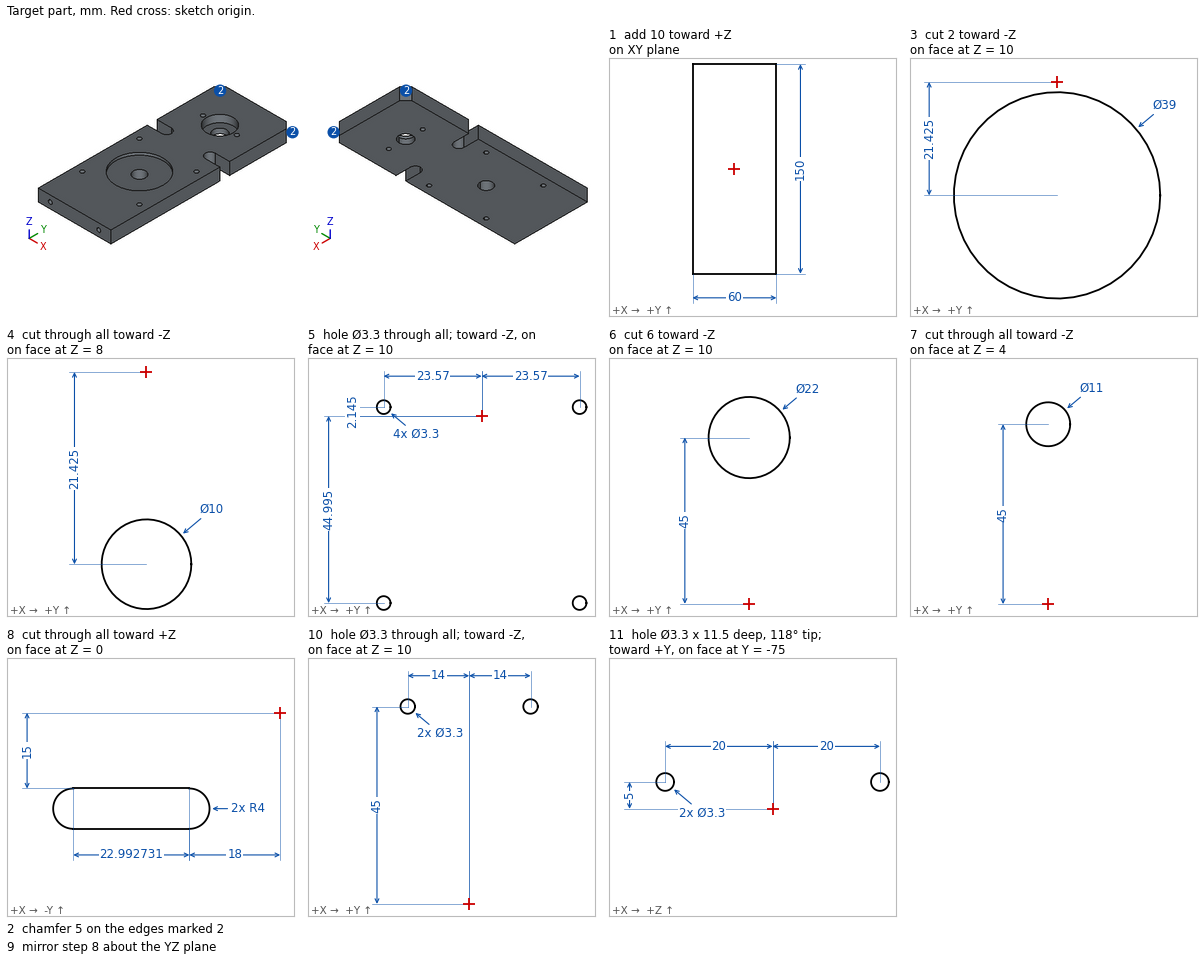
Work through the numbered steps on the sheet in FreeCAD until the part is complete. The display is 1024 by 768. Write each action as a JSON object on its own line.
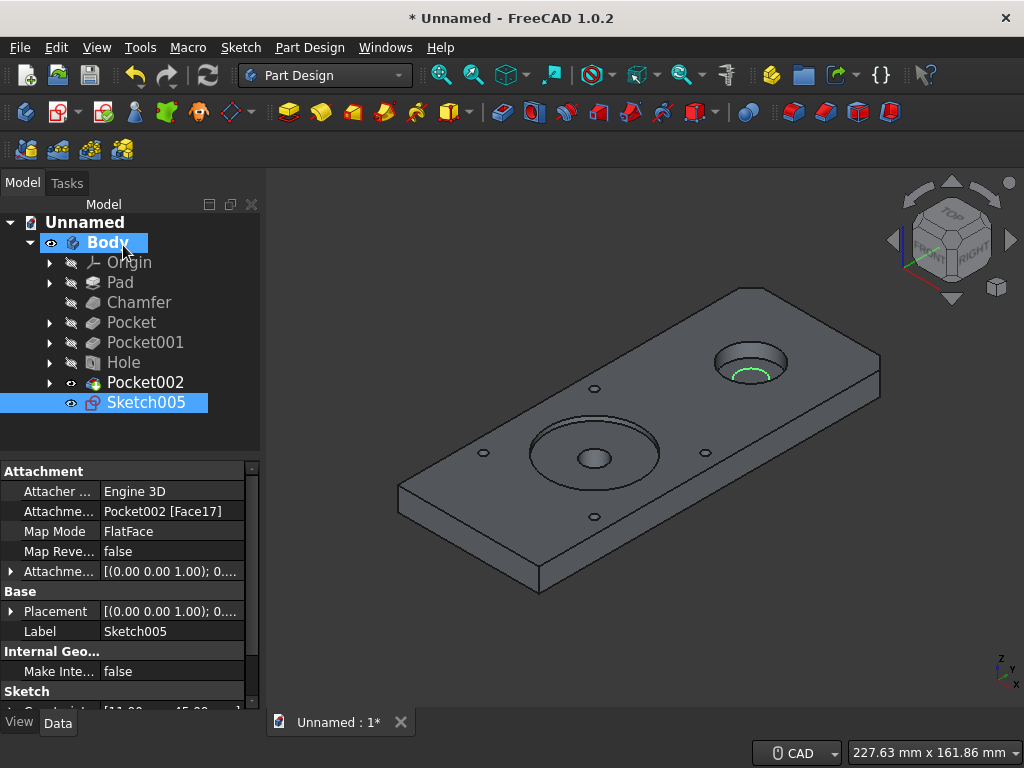
{"action": "left_click", "coordinate": [504, 112]}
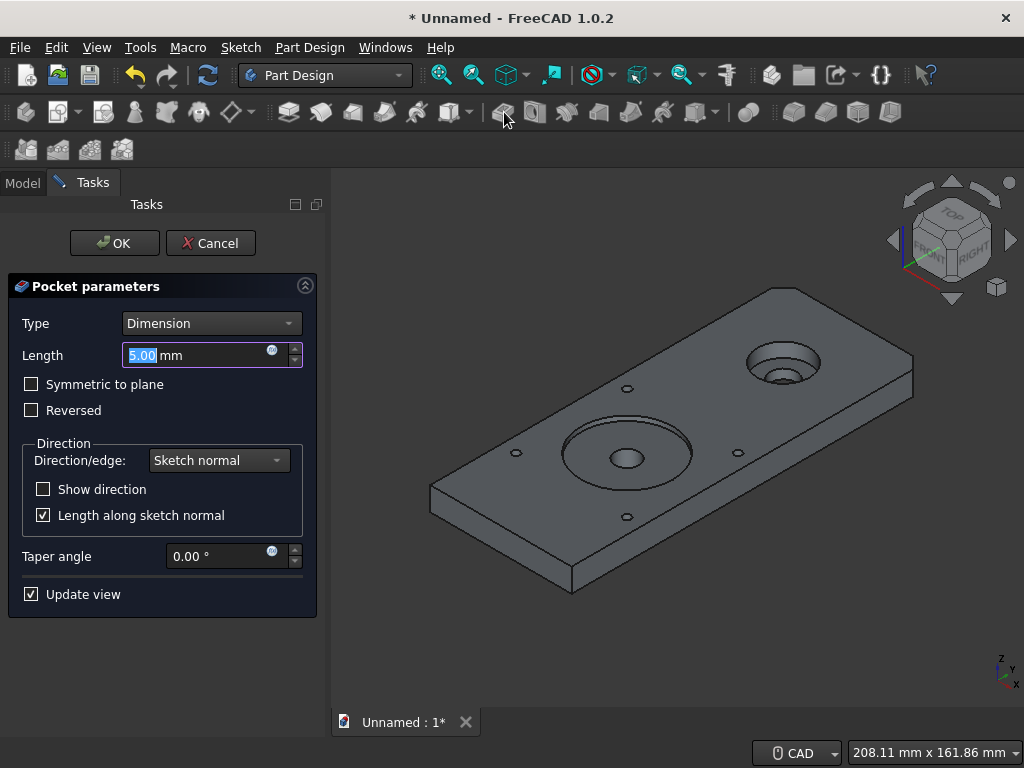
{"action": "left_click", "coordinate": [212, 324]}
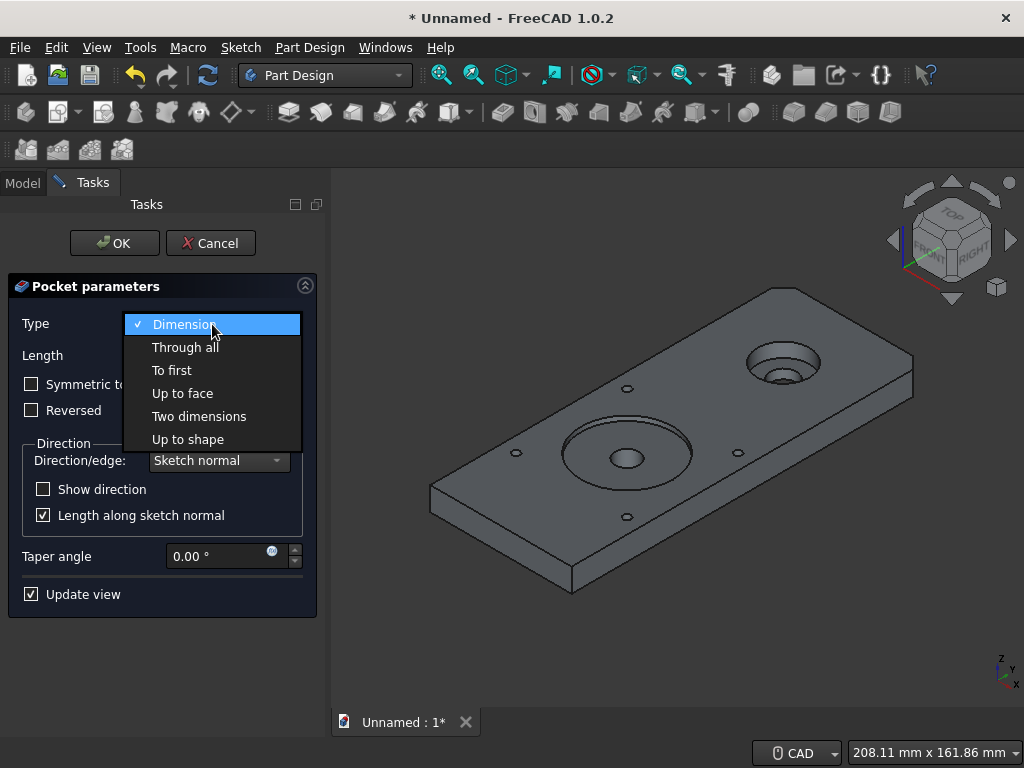
{"action": "left_click", "coordinate": [212, 348]}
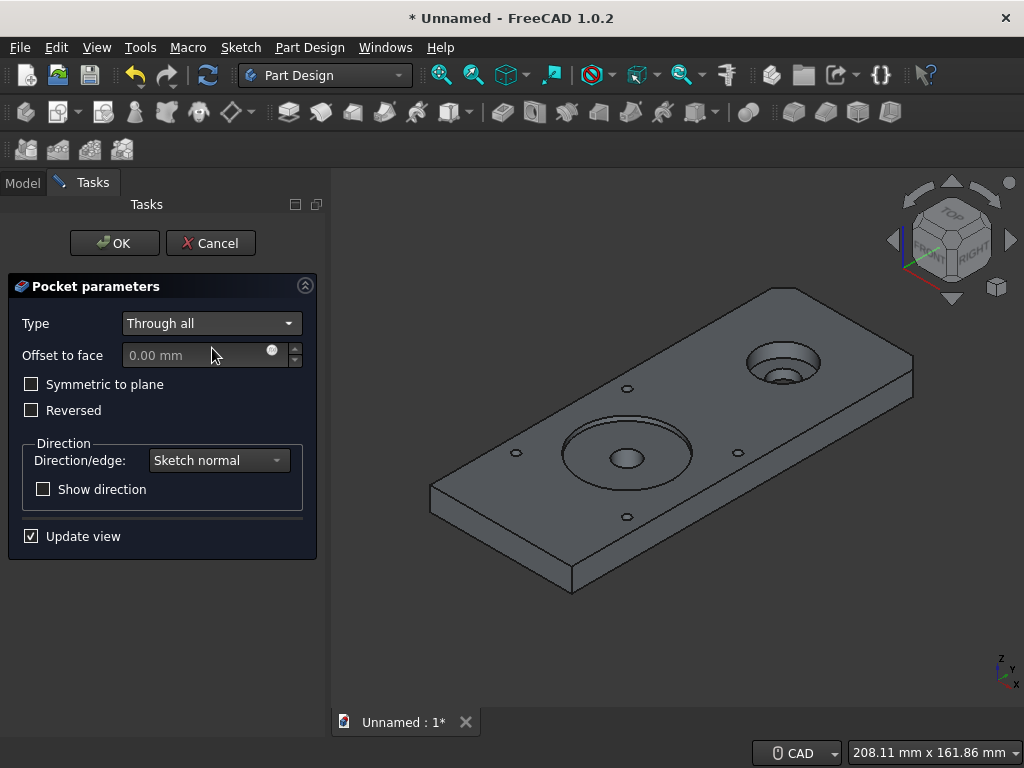
{"action": "left_click", "coordinate": [115, 243]}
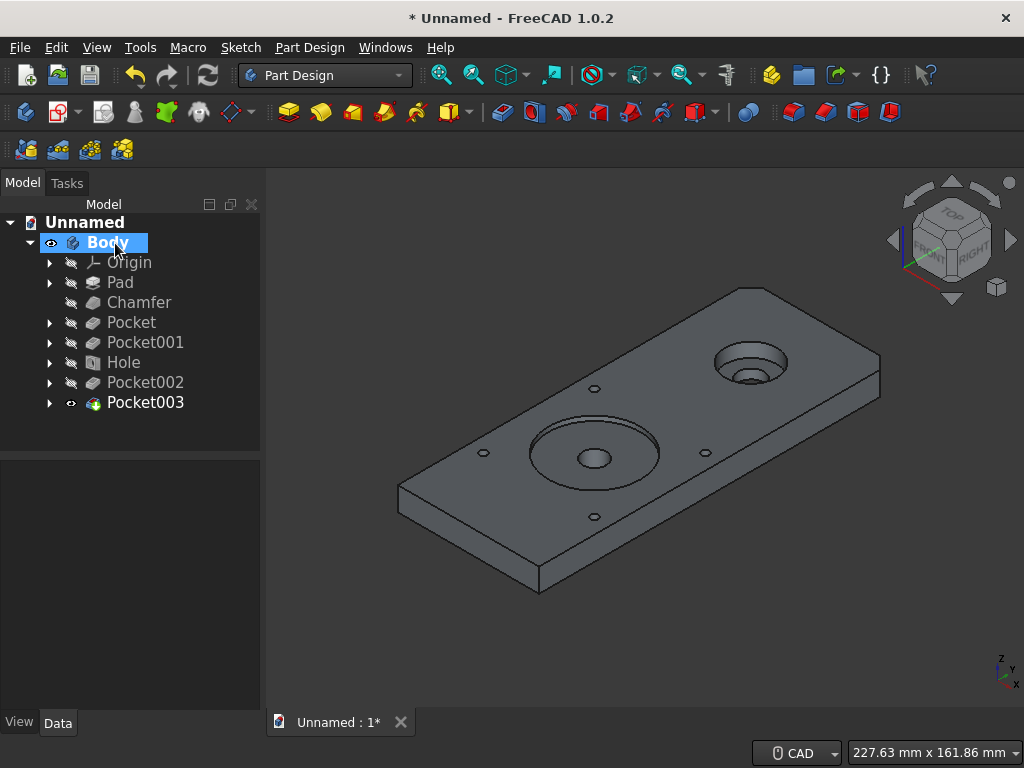
{"action": "key", "text": "5"}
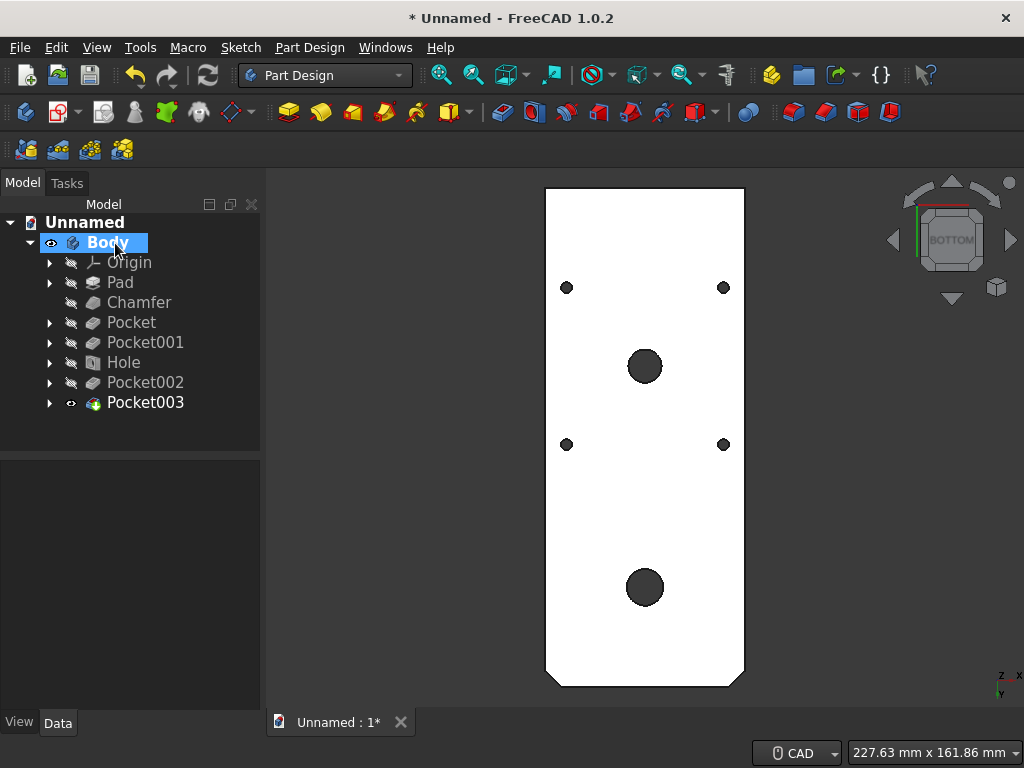
{"action": "left_click", "coordinate": [616, 508]}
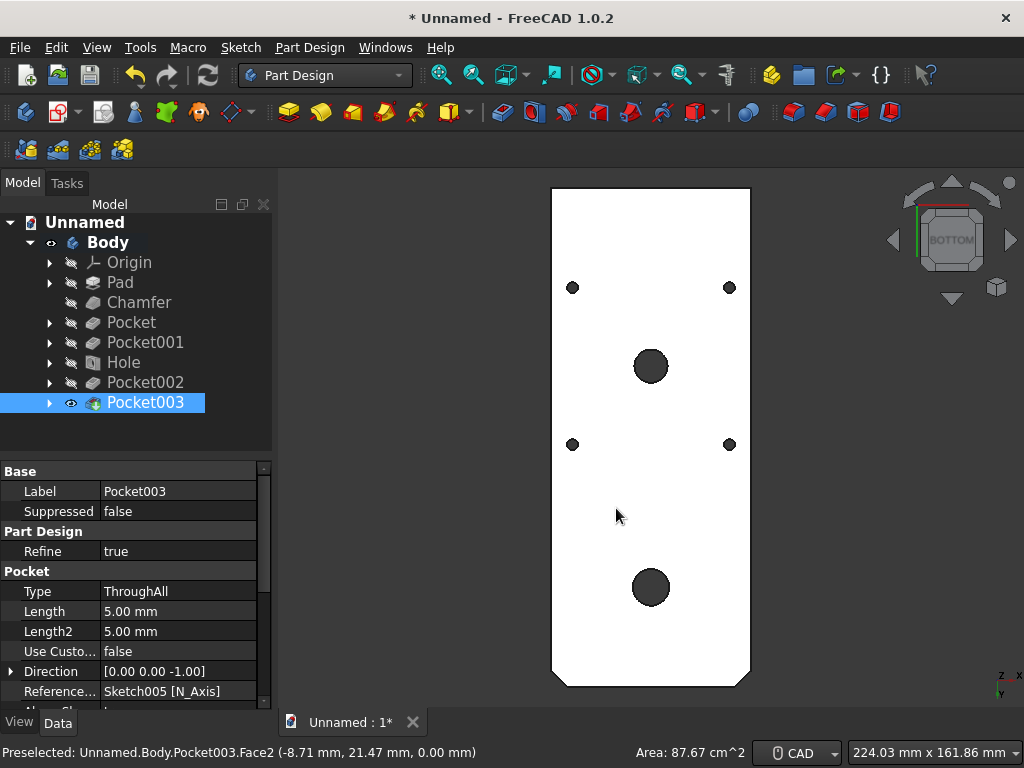
{"action": "left_click", "coordinate": [58, 112]}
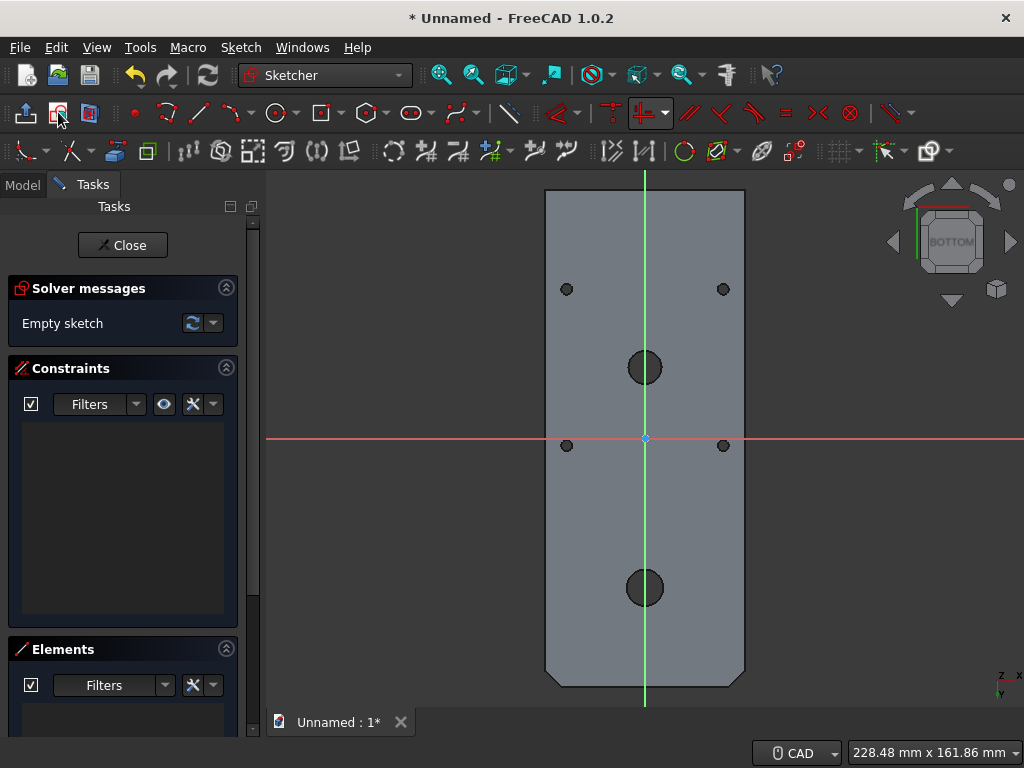
{"action": "scroll", "coordinate": [567, 499], "scroll_direction": "up", "scroll_amount": 5}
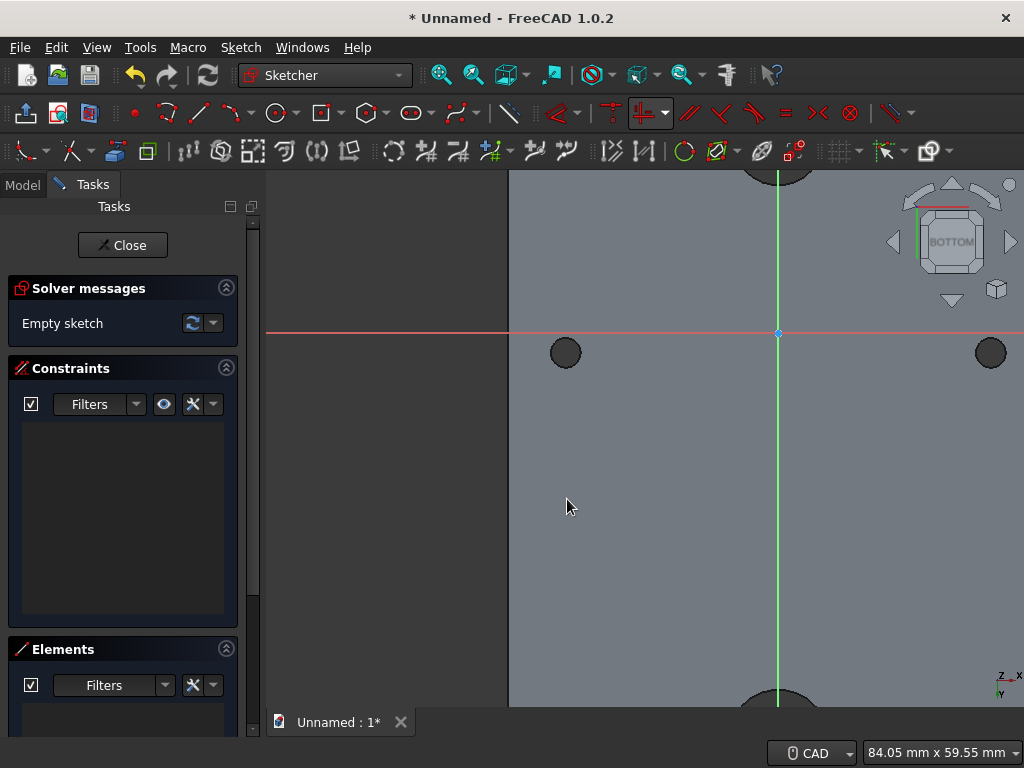
{"action": "left_click", "coordinate": [412, 114]}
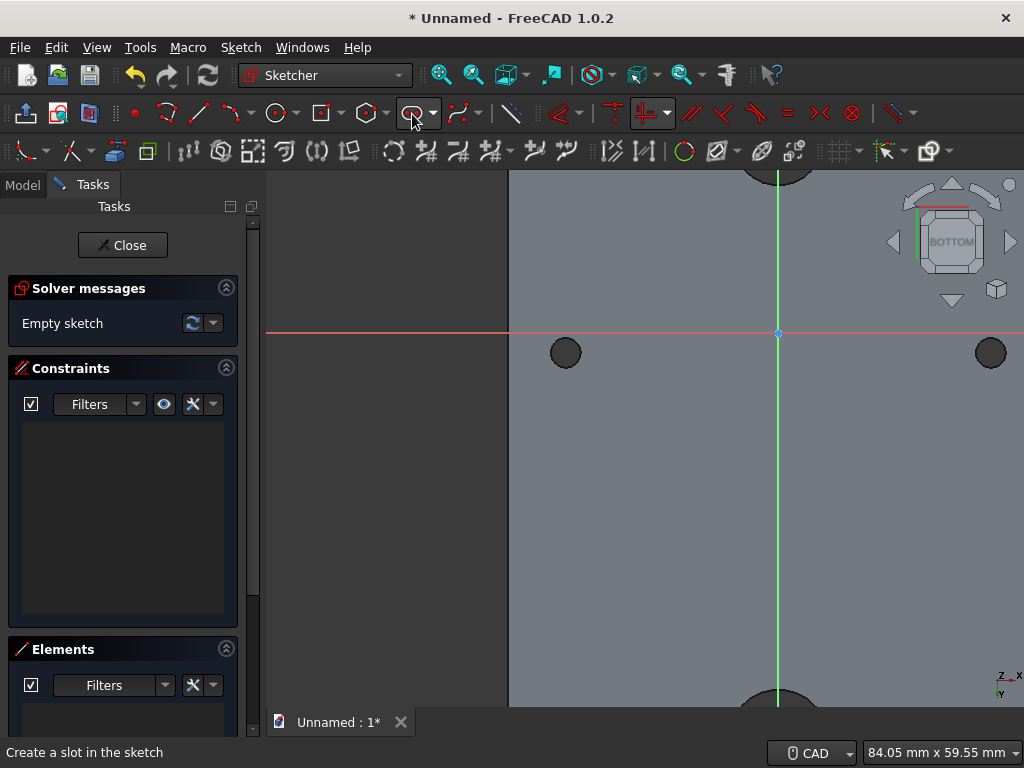
{"action": "left_click", "coordinate": [409, 505]}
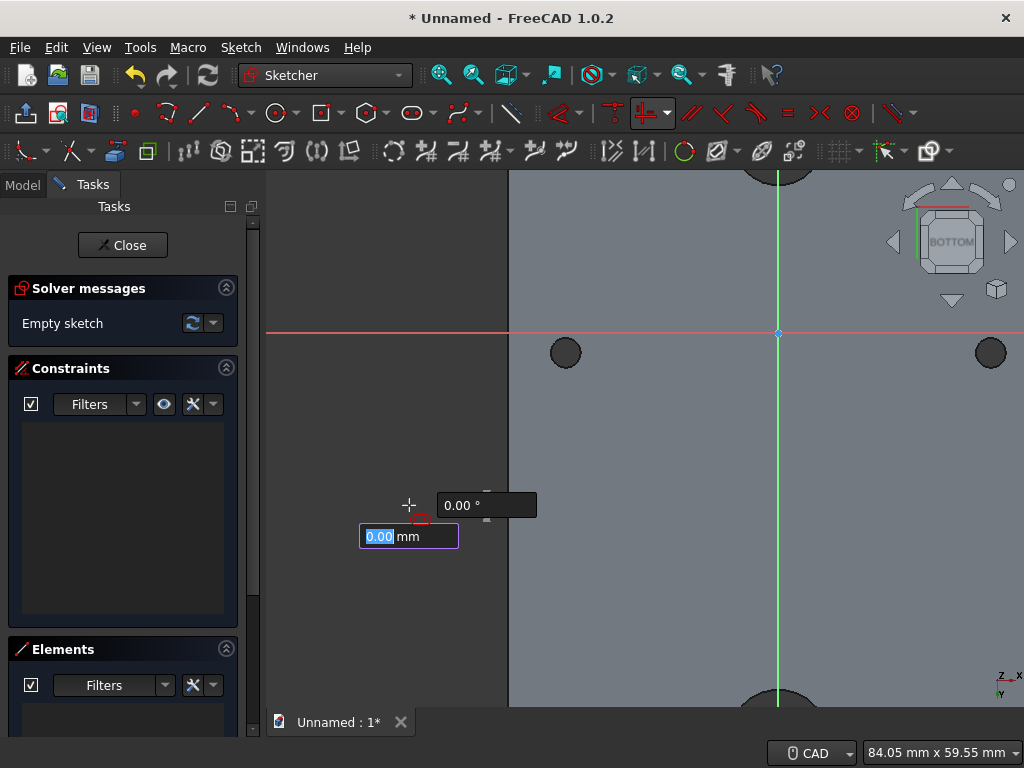
{"action": "left_click", "coordinate": [616, 505]}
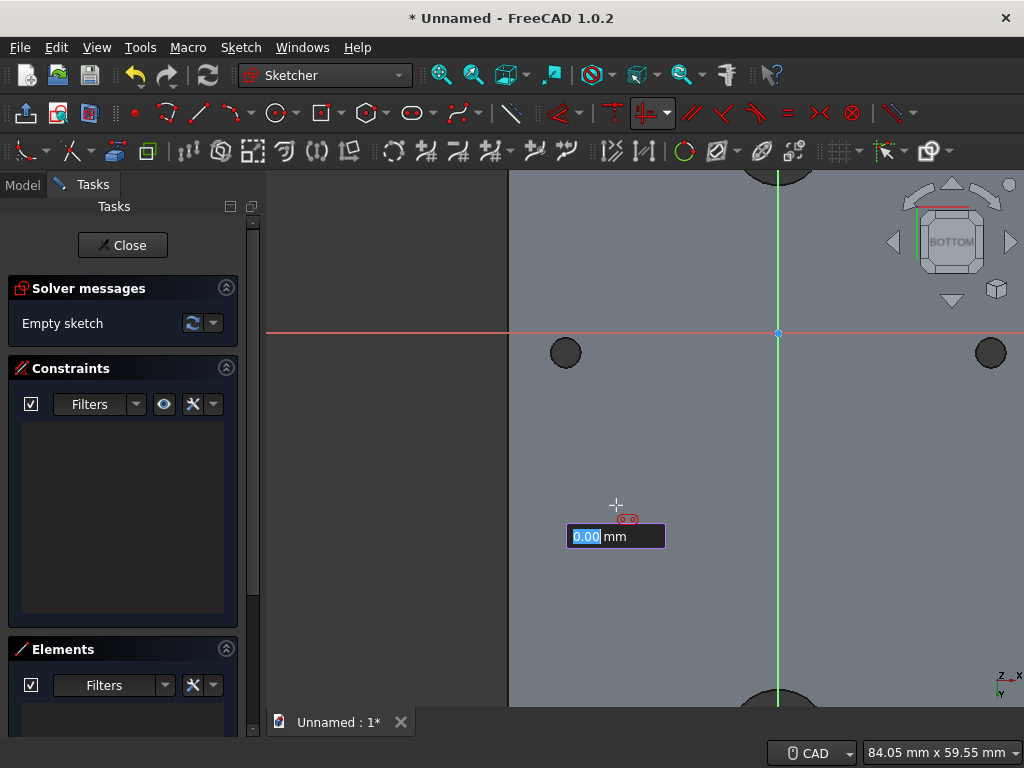
{"action": "left_click", "coordinate": [512, 541]}
{"action": "key", "text": "Escape"}